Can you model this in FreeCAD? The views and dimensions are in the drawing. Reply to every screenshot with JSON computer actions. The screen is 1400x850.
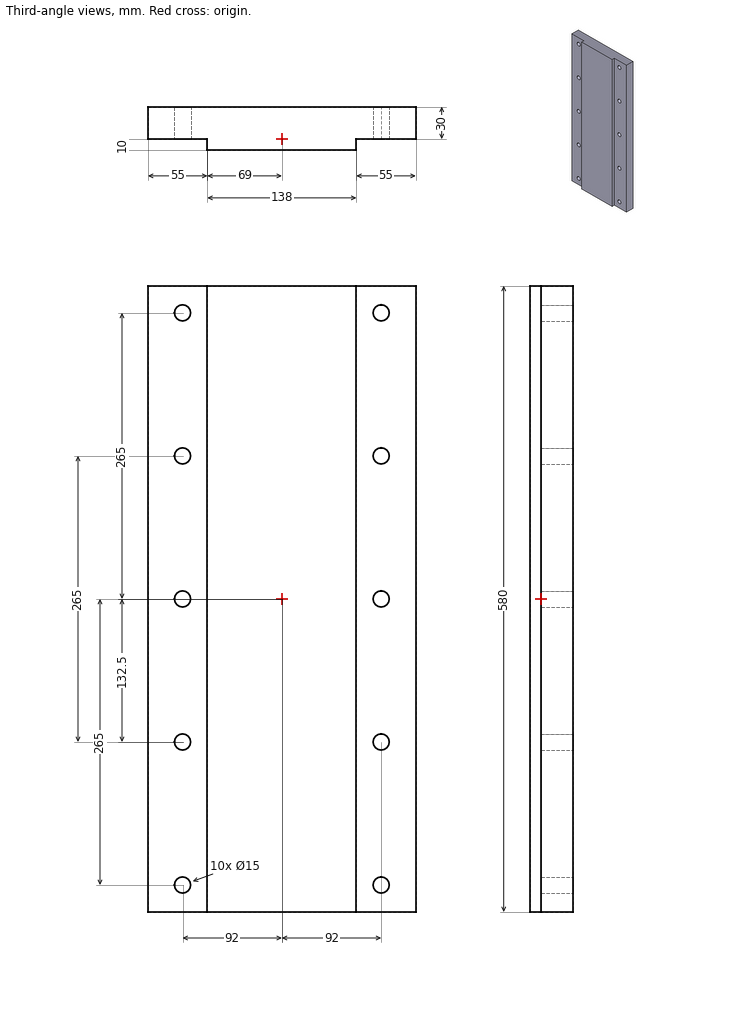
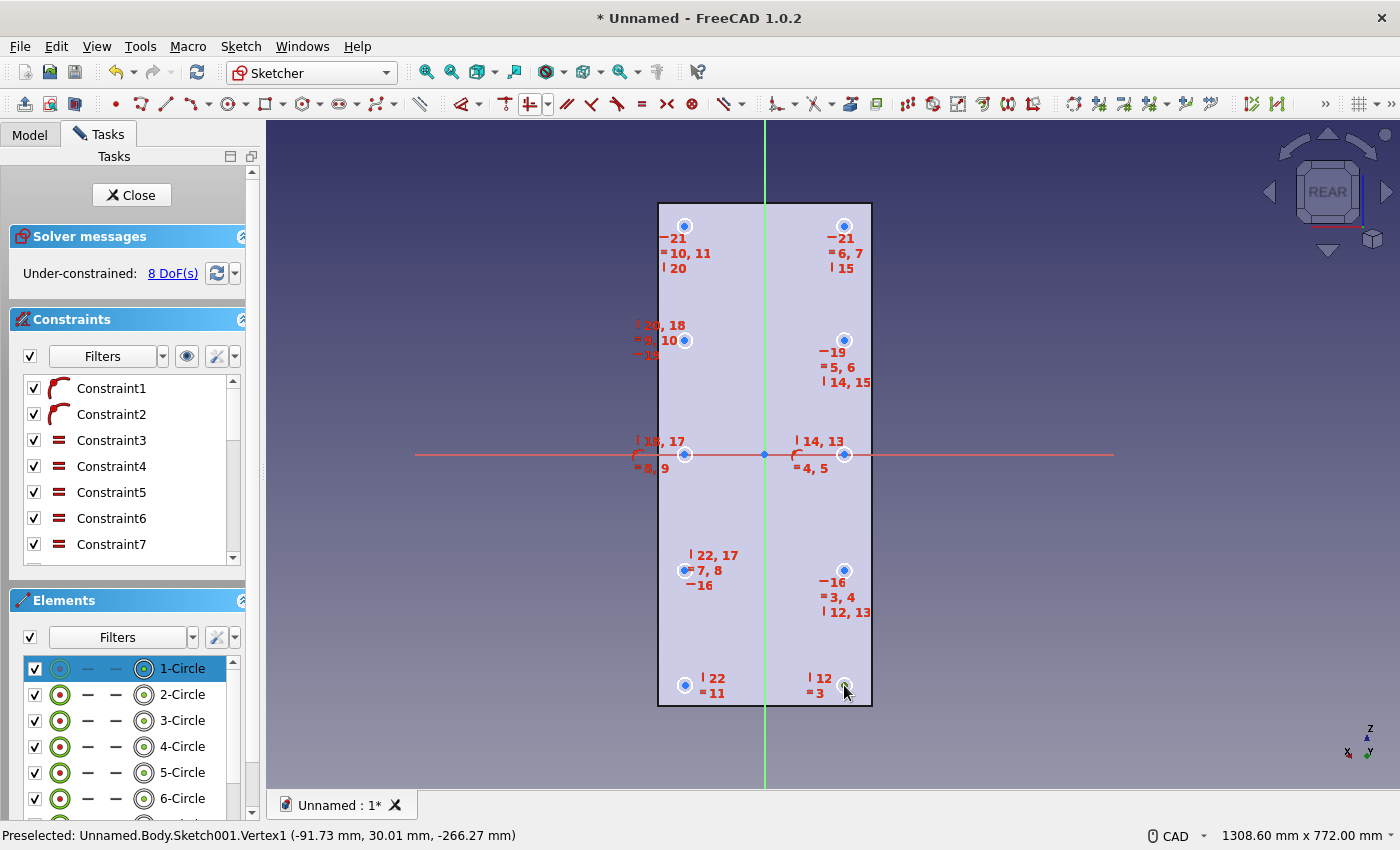
{"action": "left_click", "coordinate": [685, 685]}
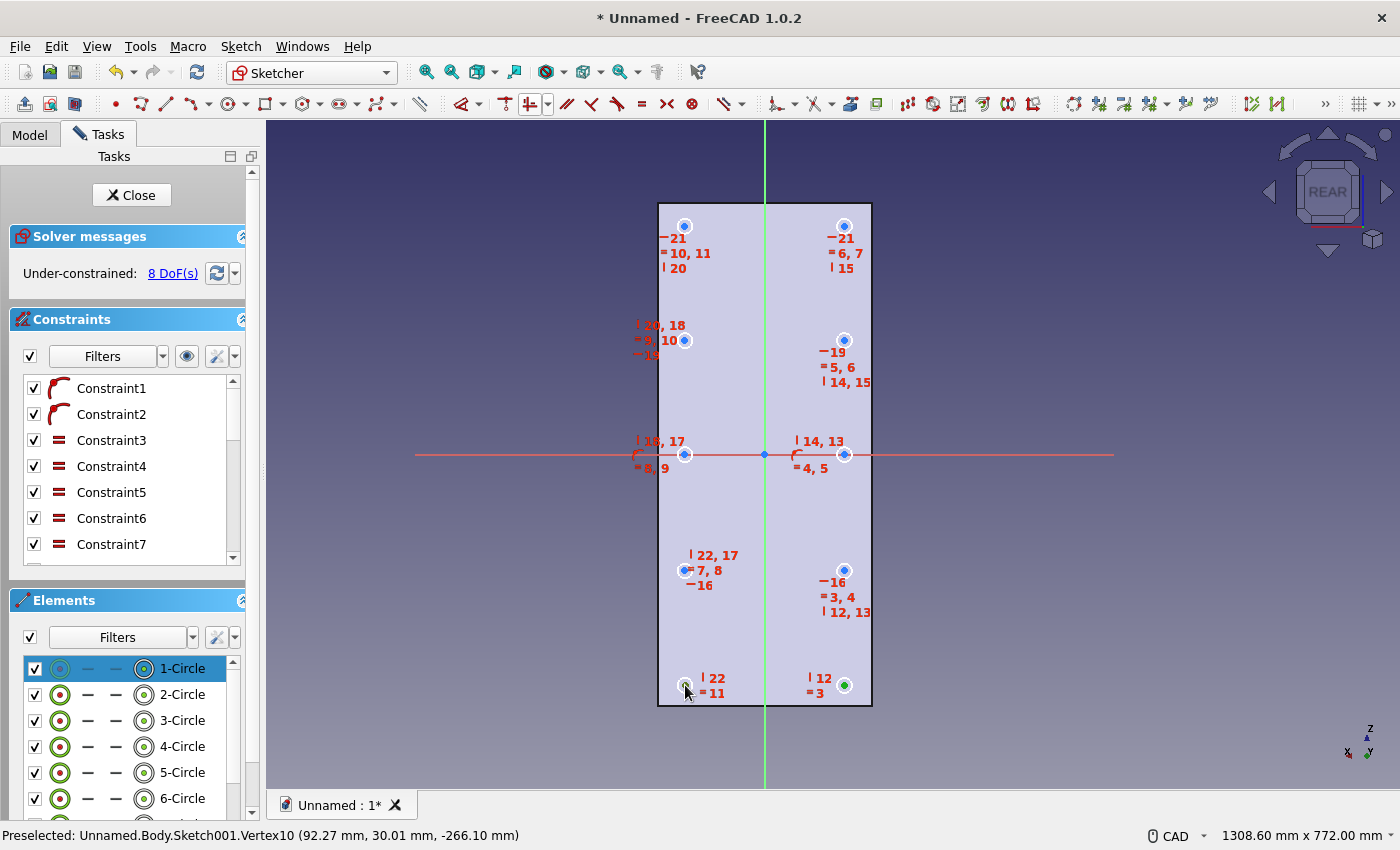
{"action": "left_click", "coordinate": [548, 104]}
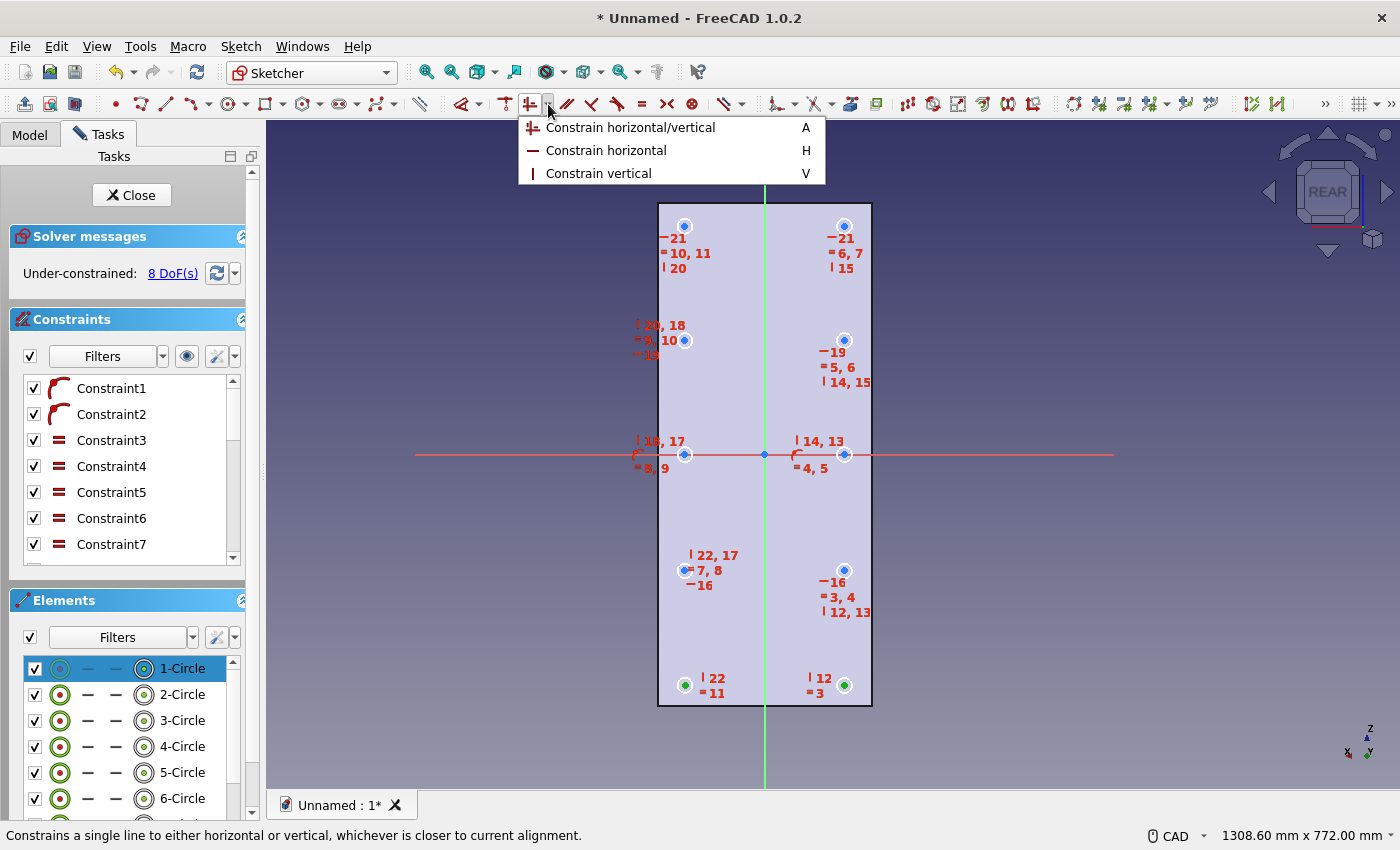
{"action": "left_click", "coordinate": [672, 150]}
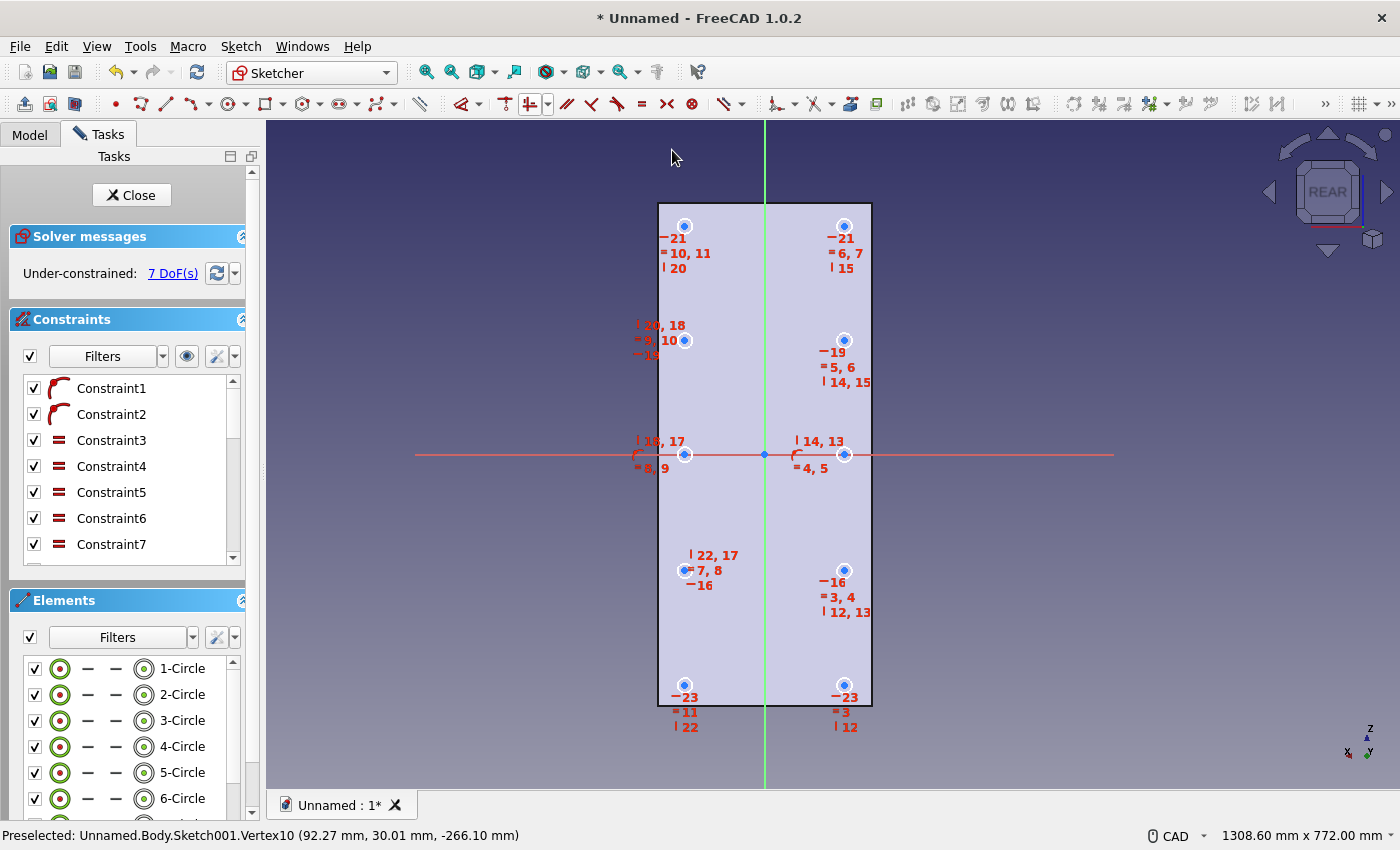
{"action": "key", "text": "d"}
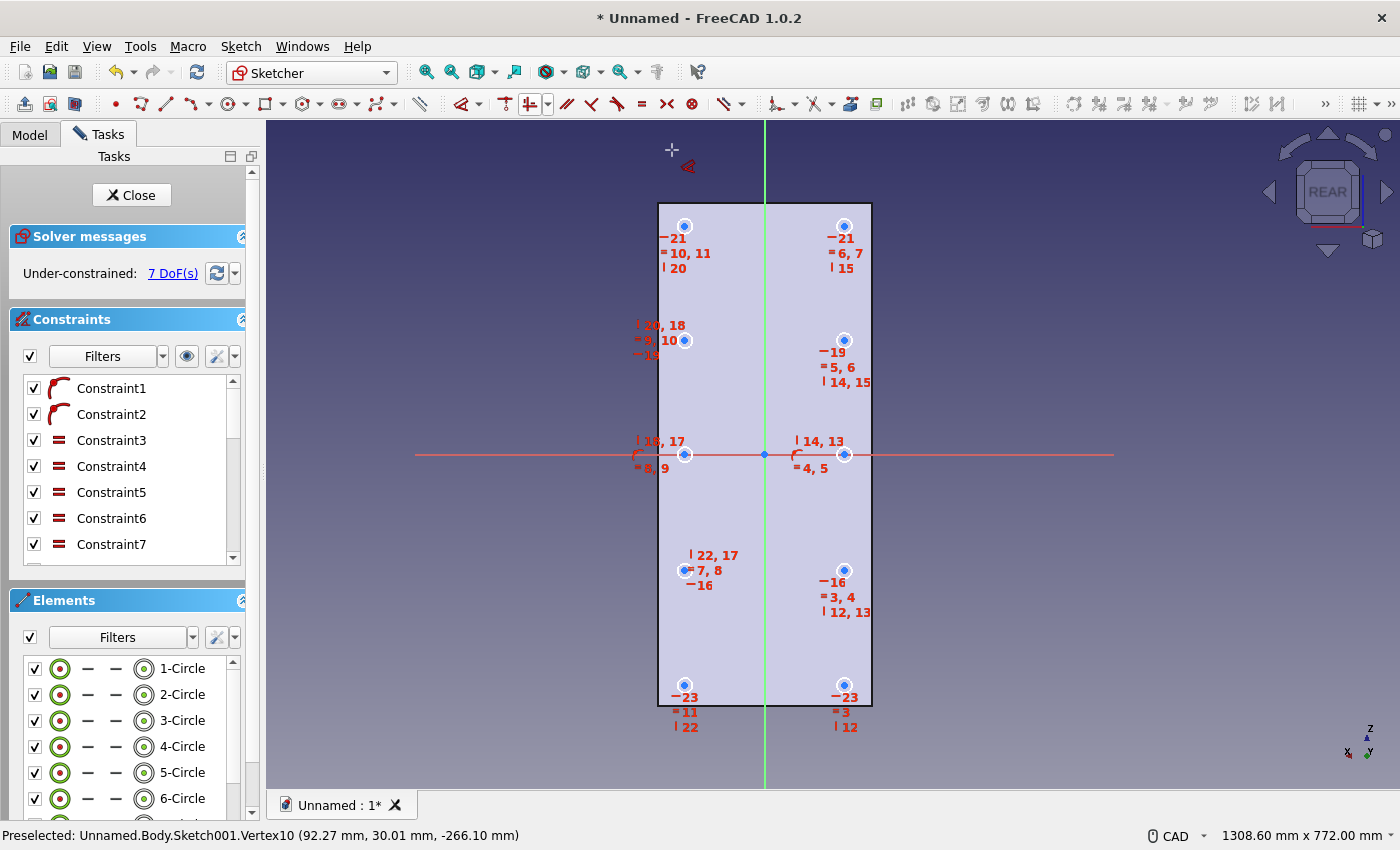
{"action": "scroll", "coordinate": [850, 680], "scroll_direction": "up", "scroll_amount": 6}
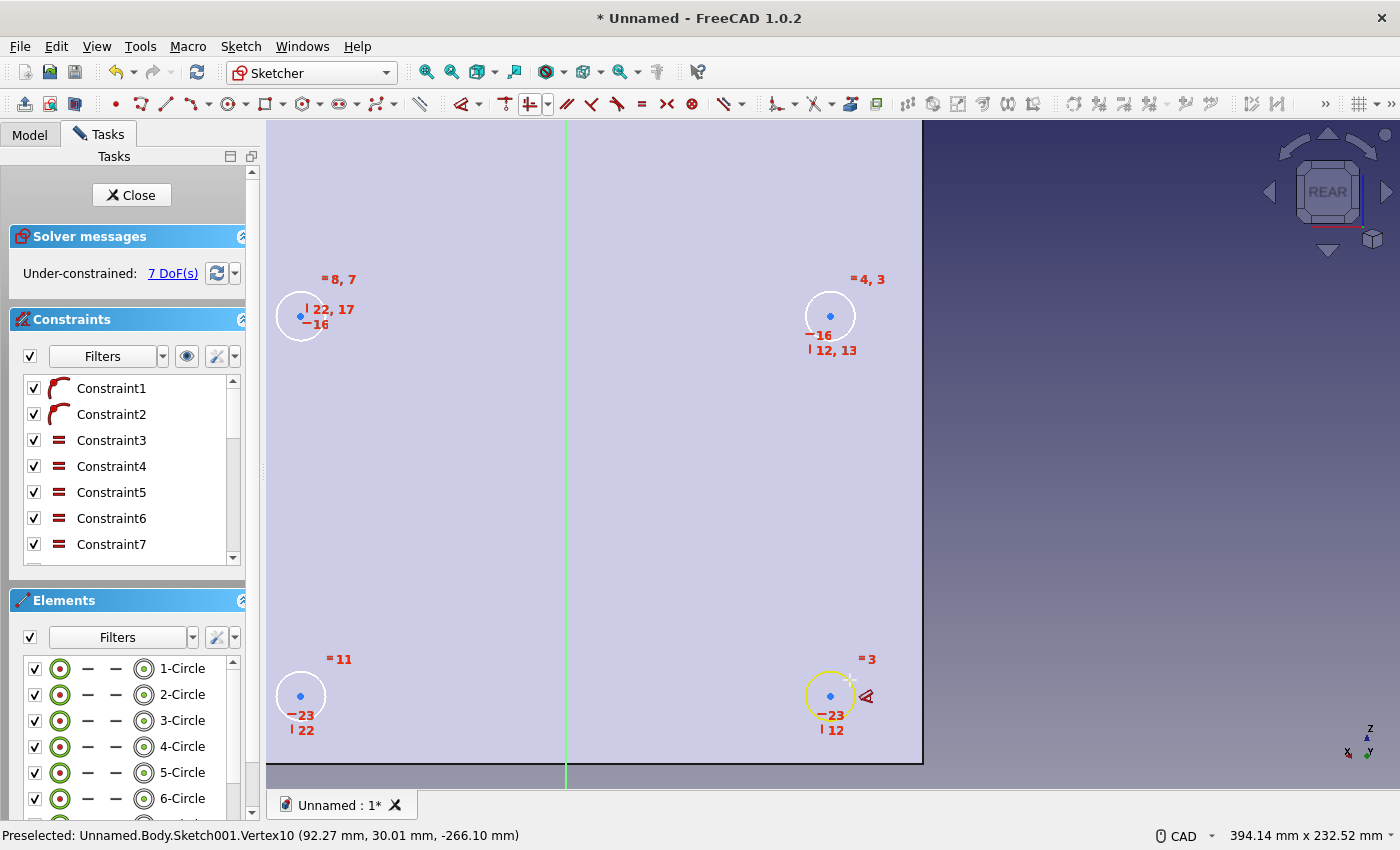
{"action": "left_click", "coordinate": [848, 679]}
{"action": "left_click", "coordinate": [871, 657]}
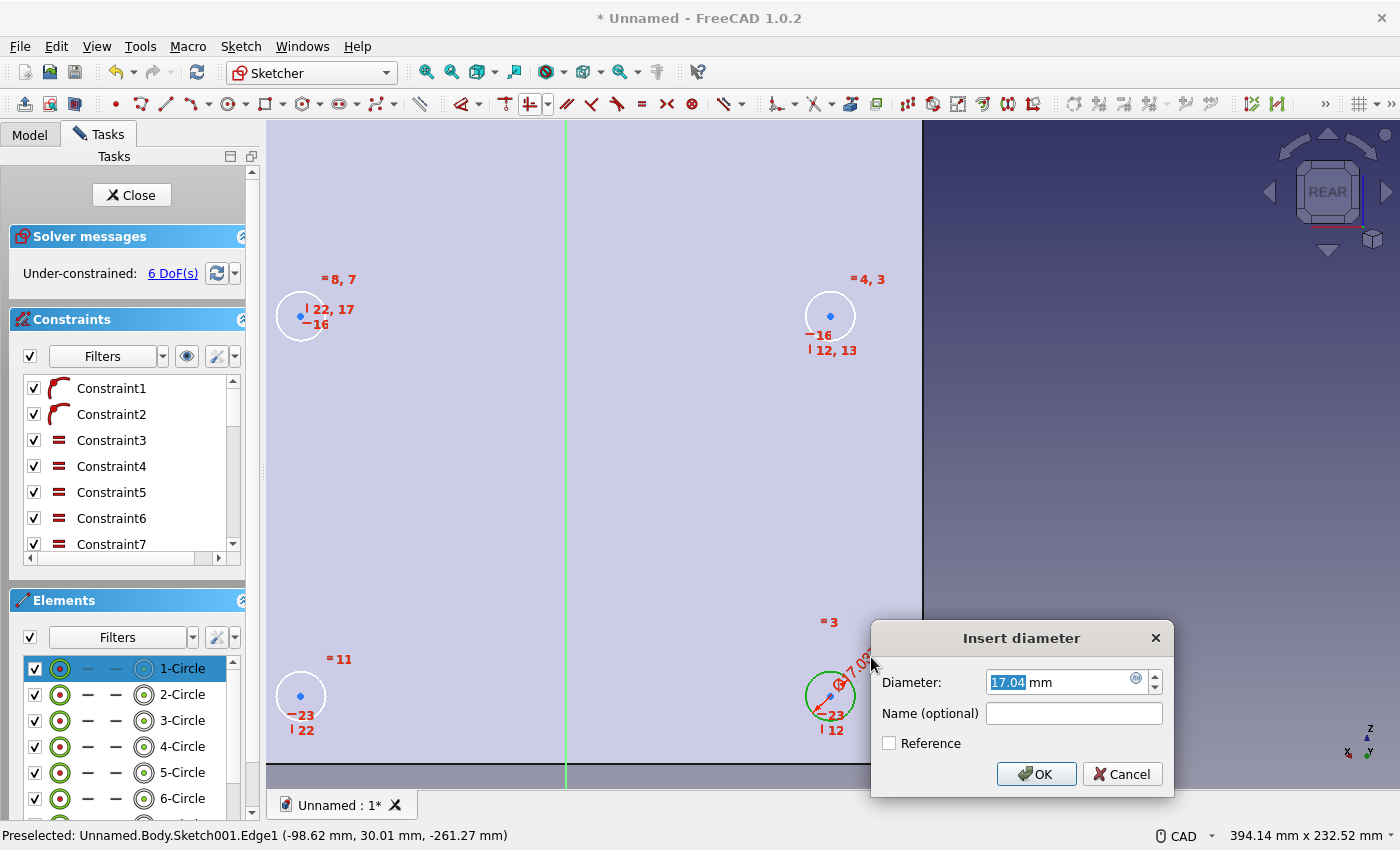
{"action": "type", "text": "15"}
{"action": "key", "text": "Return"}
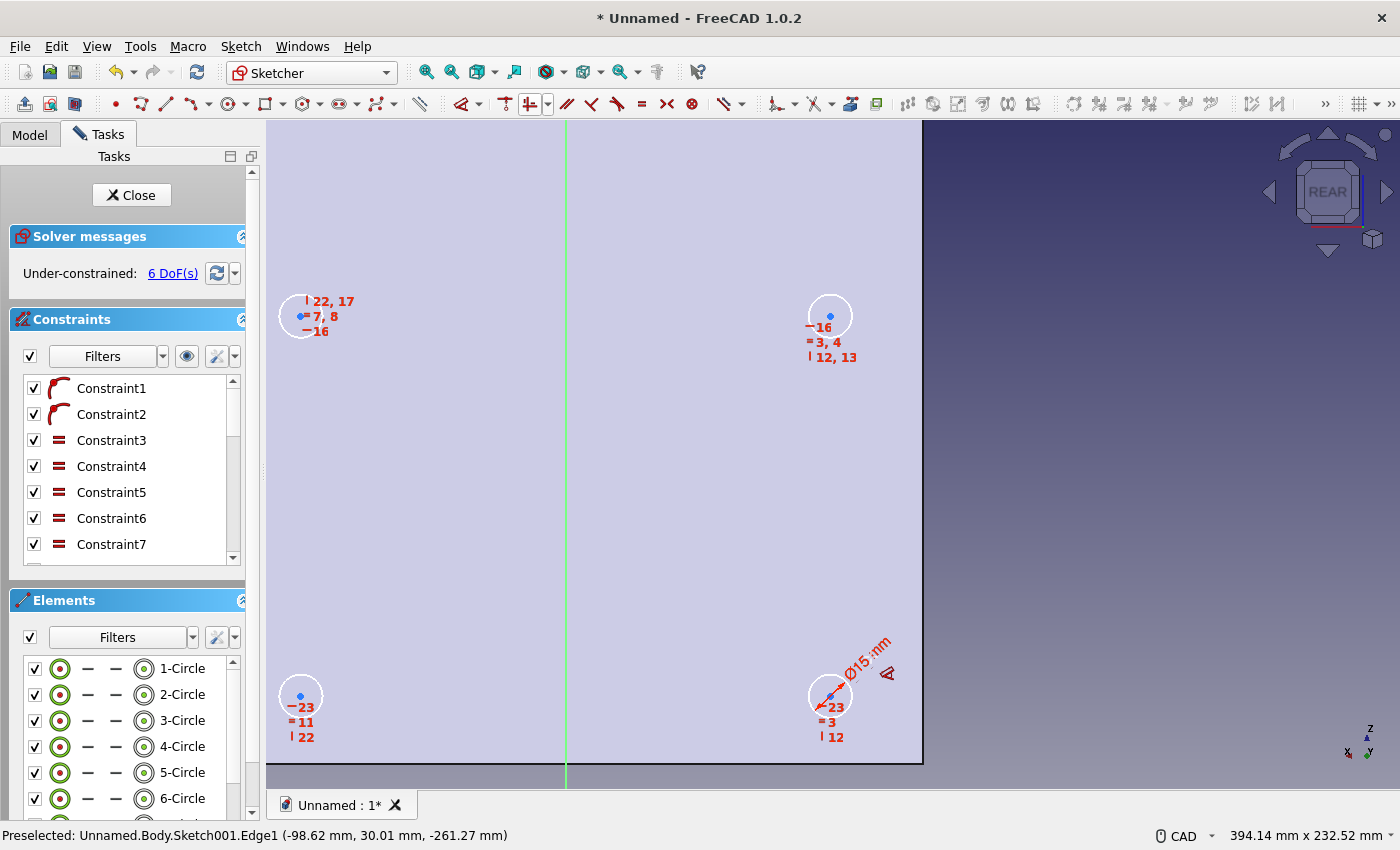
{"action": "left_click", "coordinate": [830, 696]}
{"action": "left_click", "coordinate": [698, 730]}